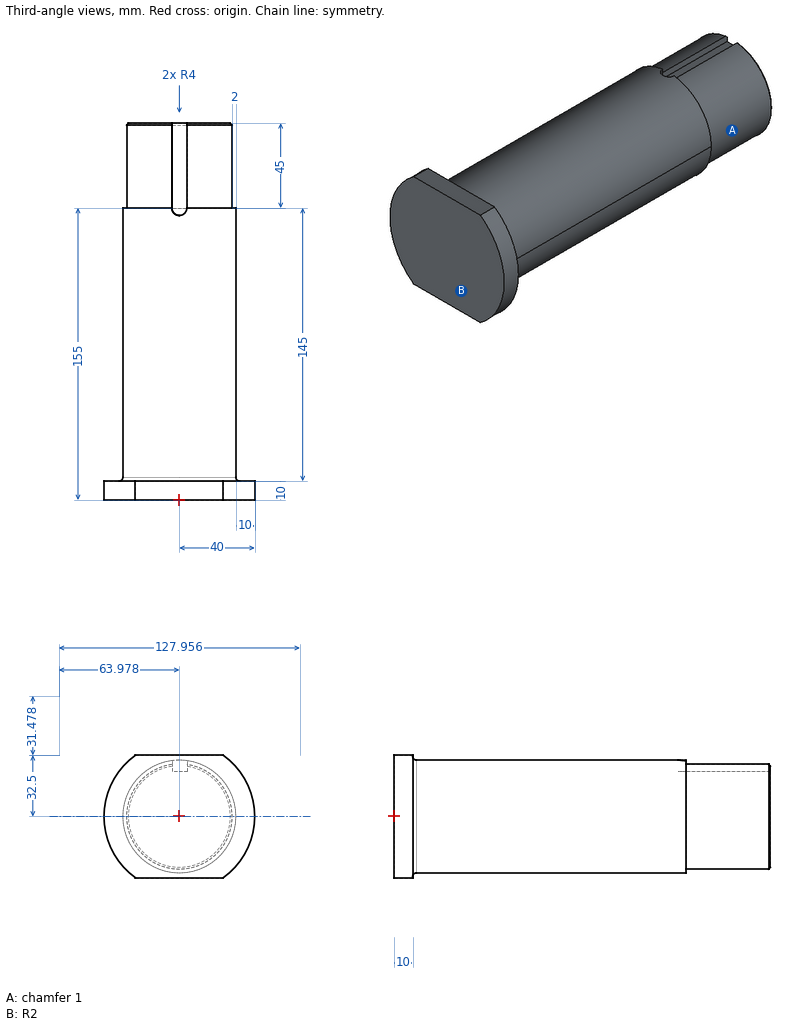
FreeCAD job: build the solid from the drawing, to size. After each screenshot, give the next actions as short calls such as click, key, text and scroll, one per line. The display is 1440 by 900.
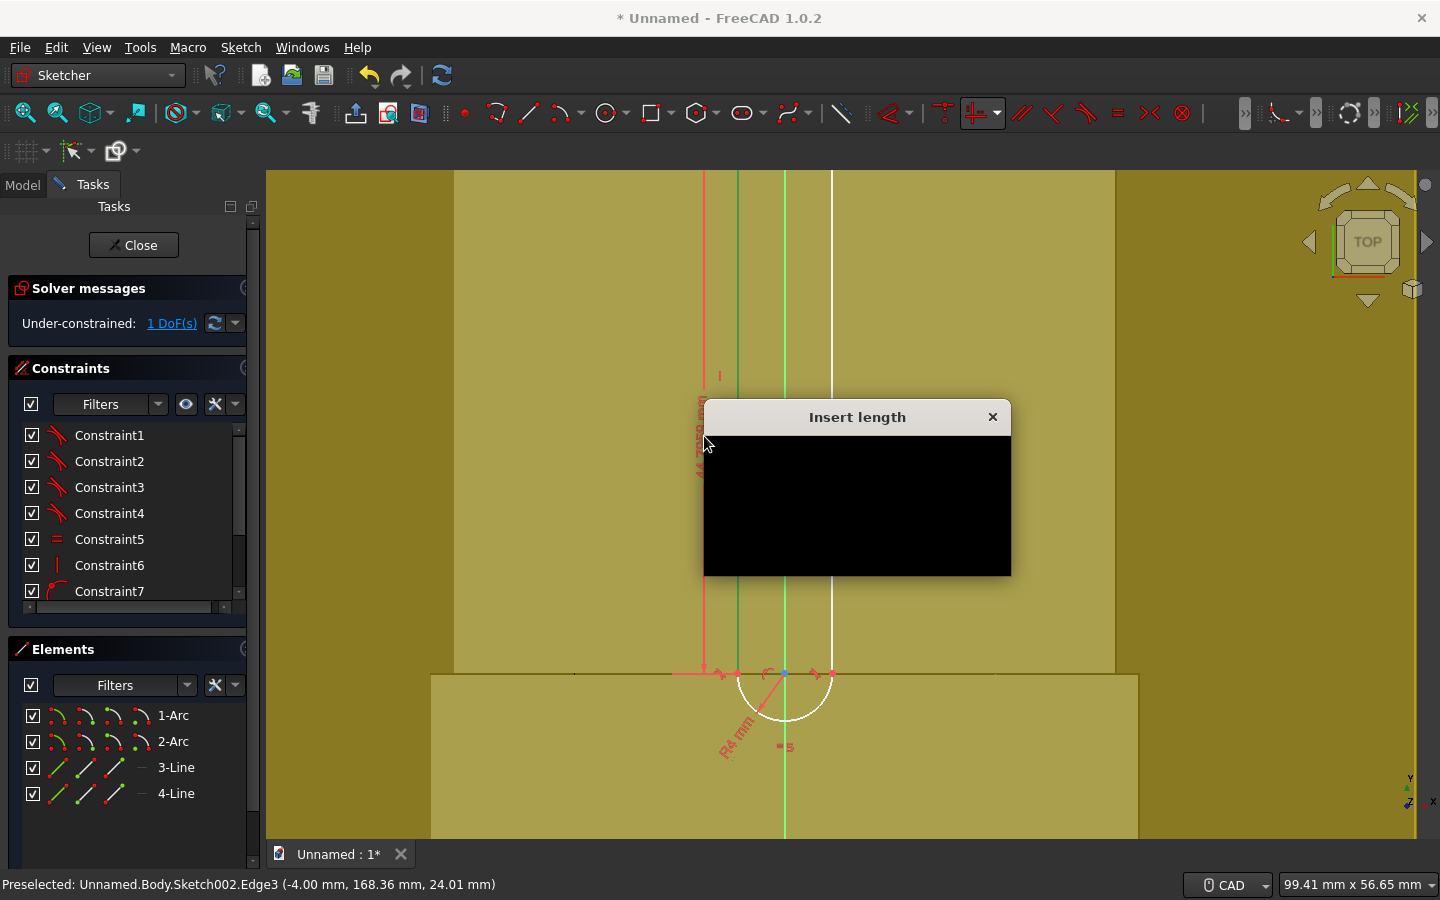
text(45)
key(Return)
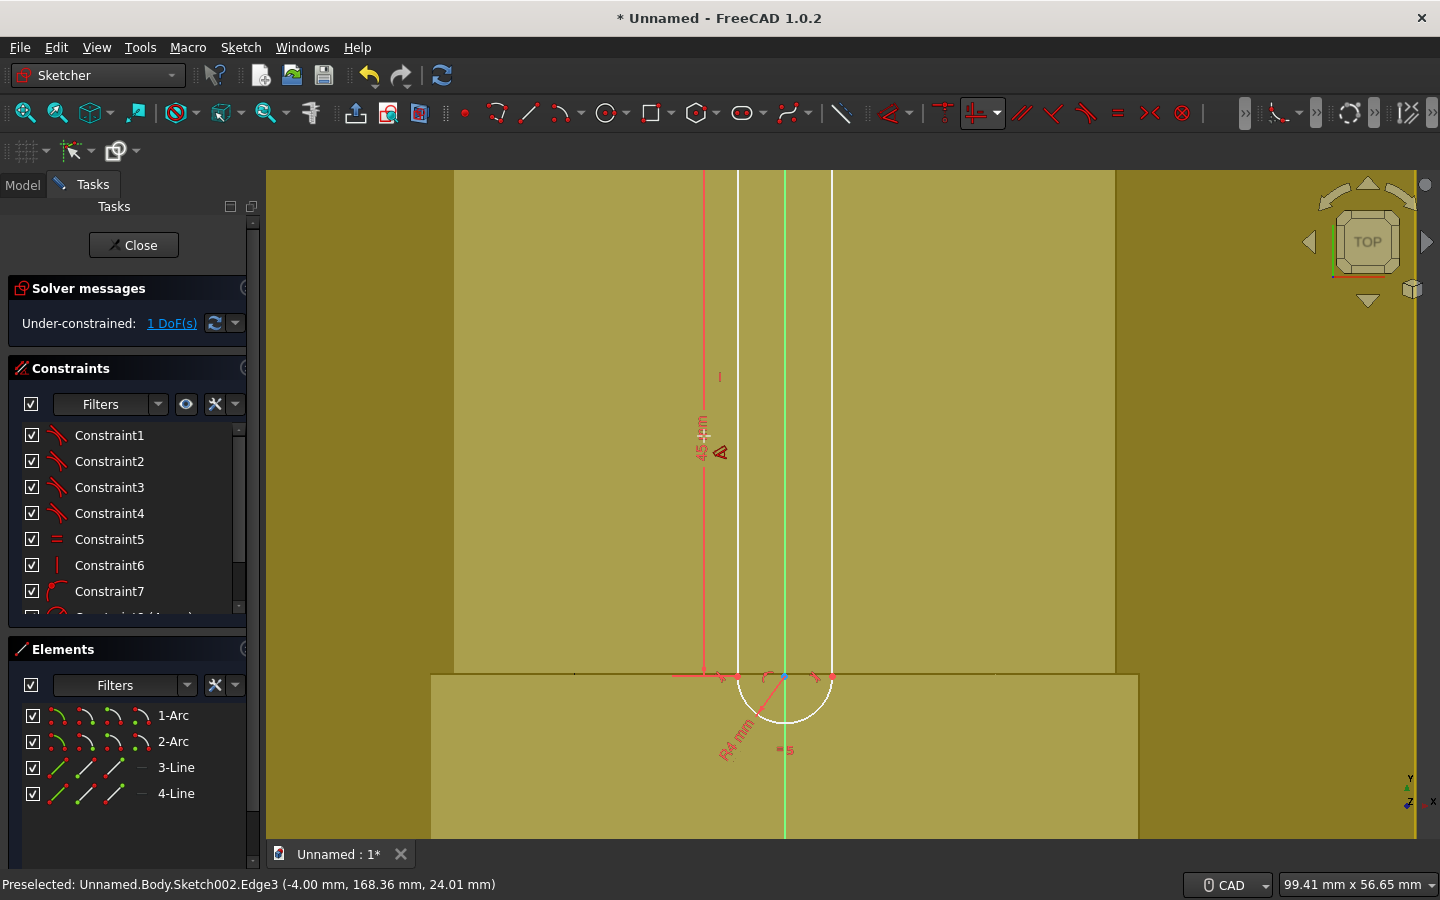
click(738, 676)
click(704, 775)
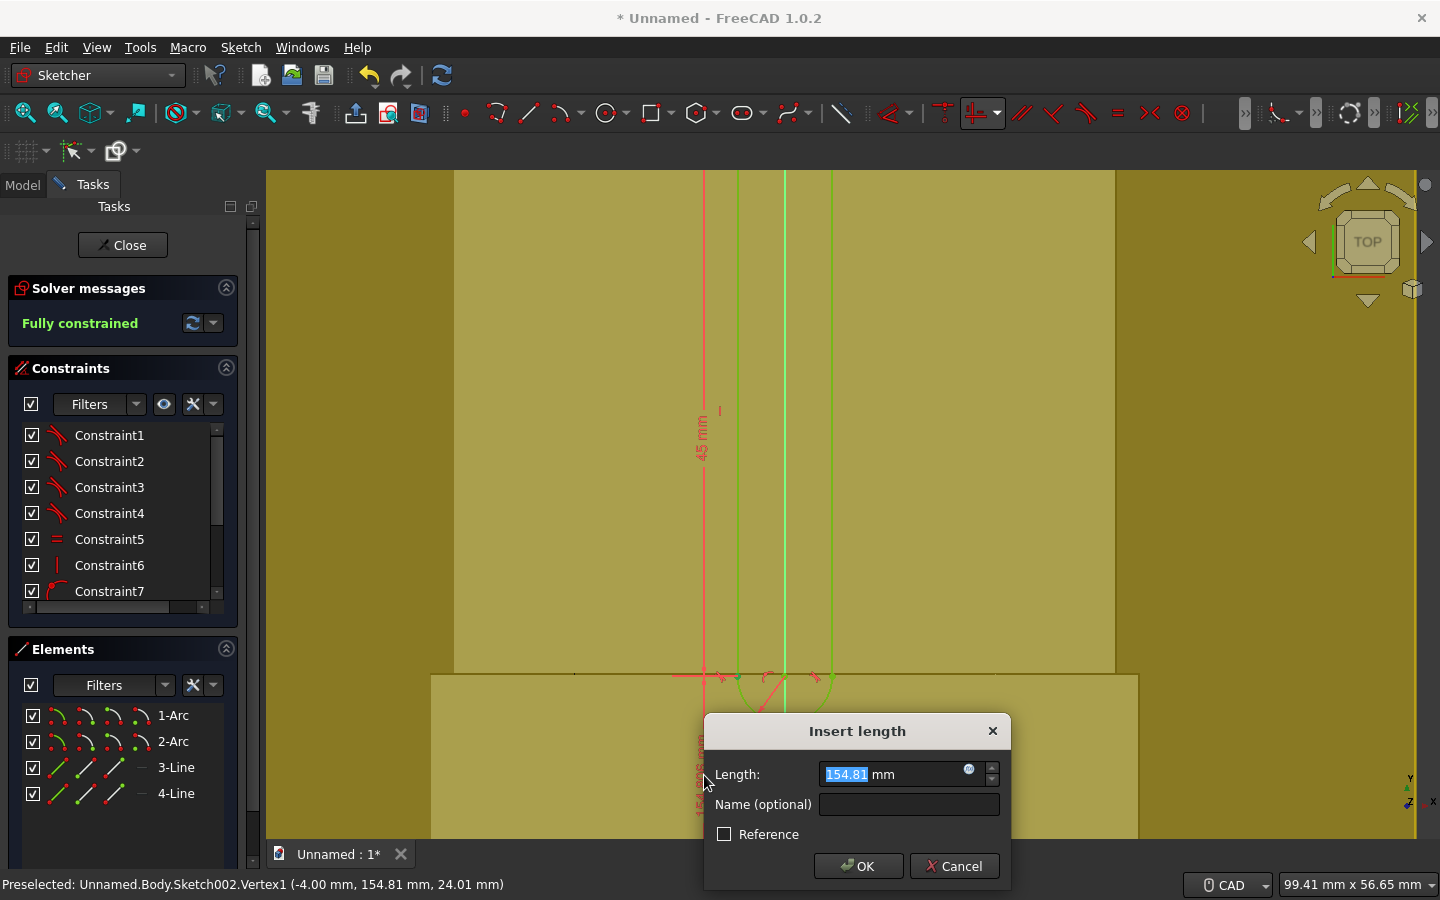
text(155)
key(Return)
key(Escape)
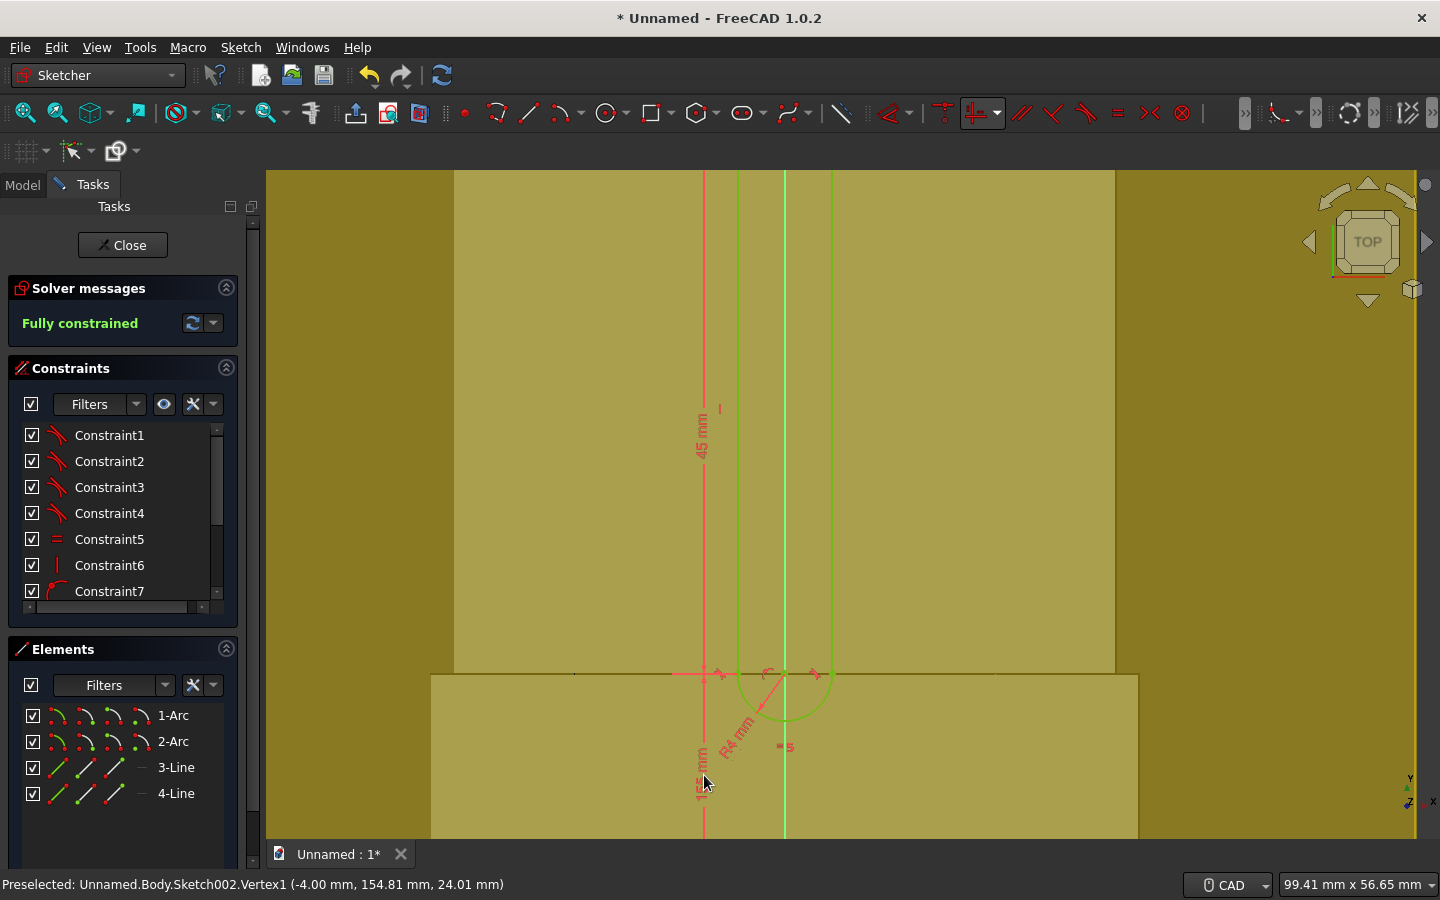
click(123, 245)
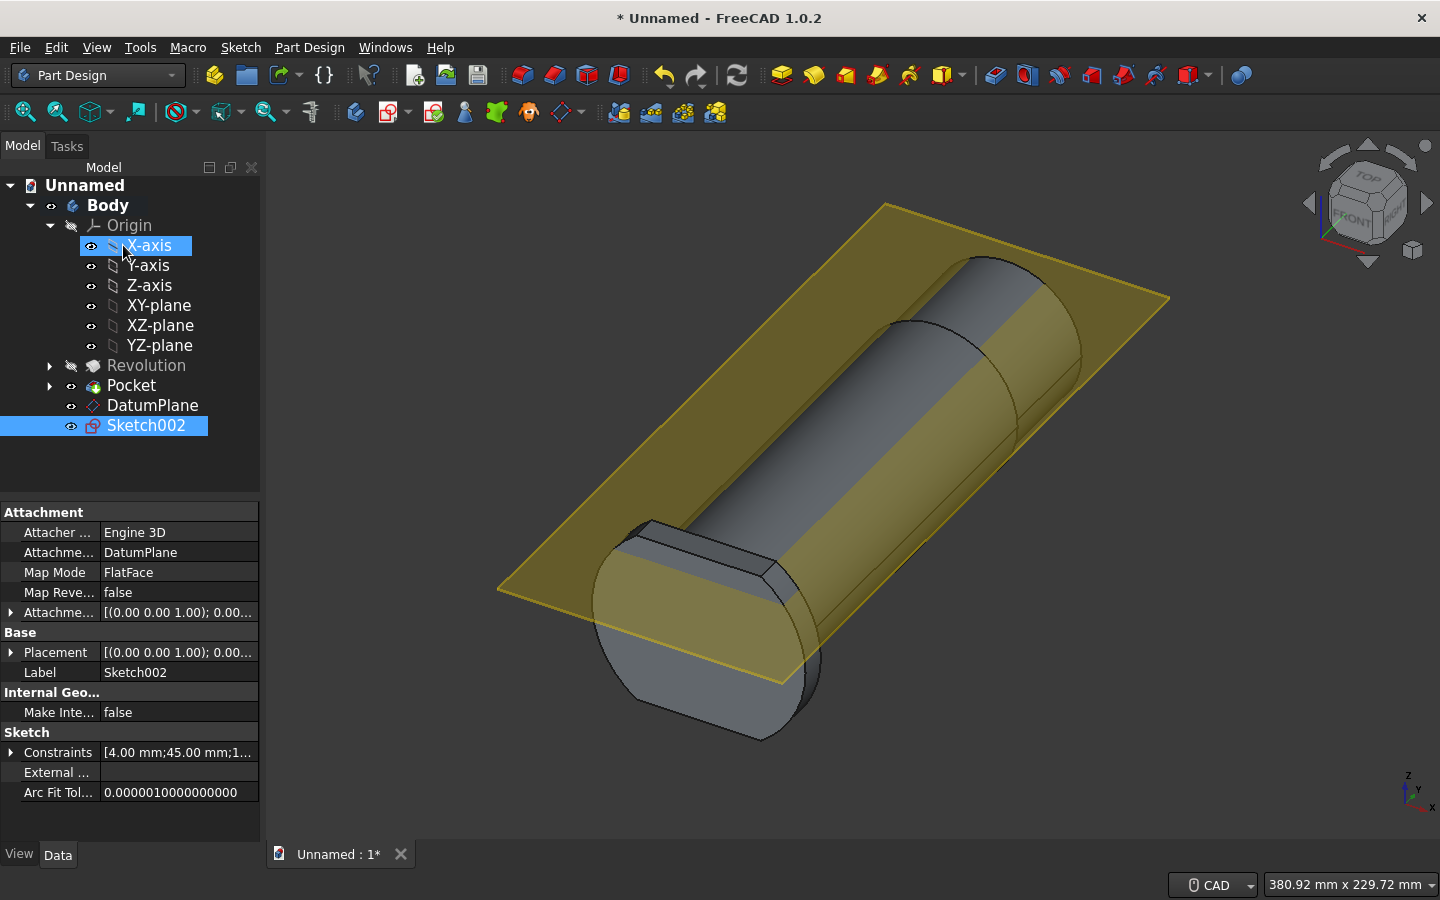
click(996, 76)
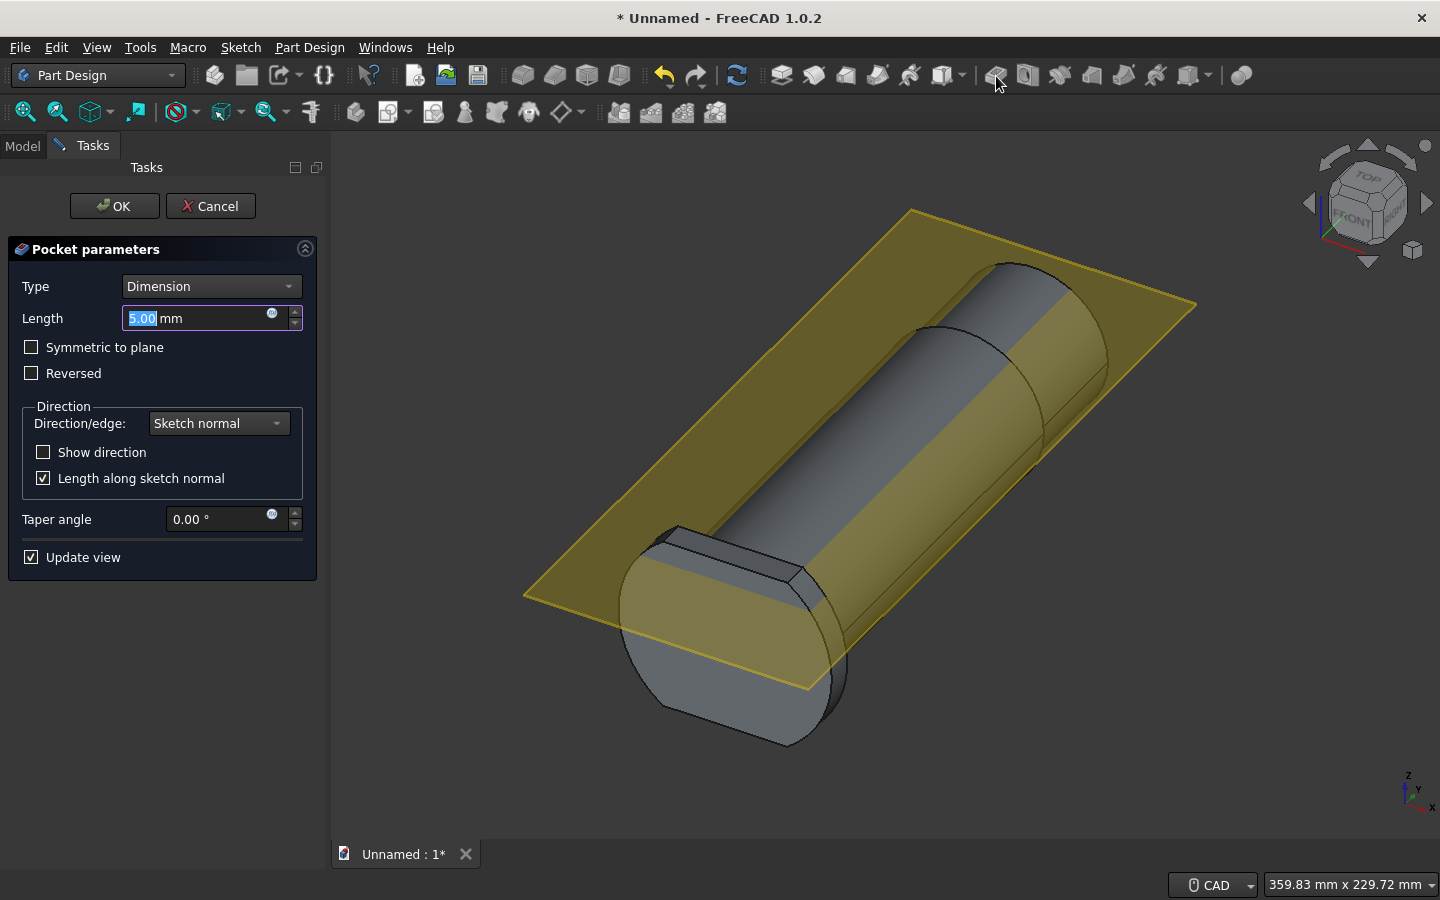
click(212, 286)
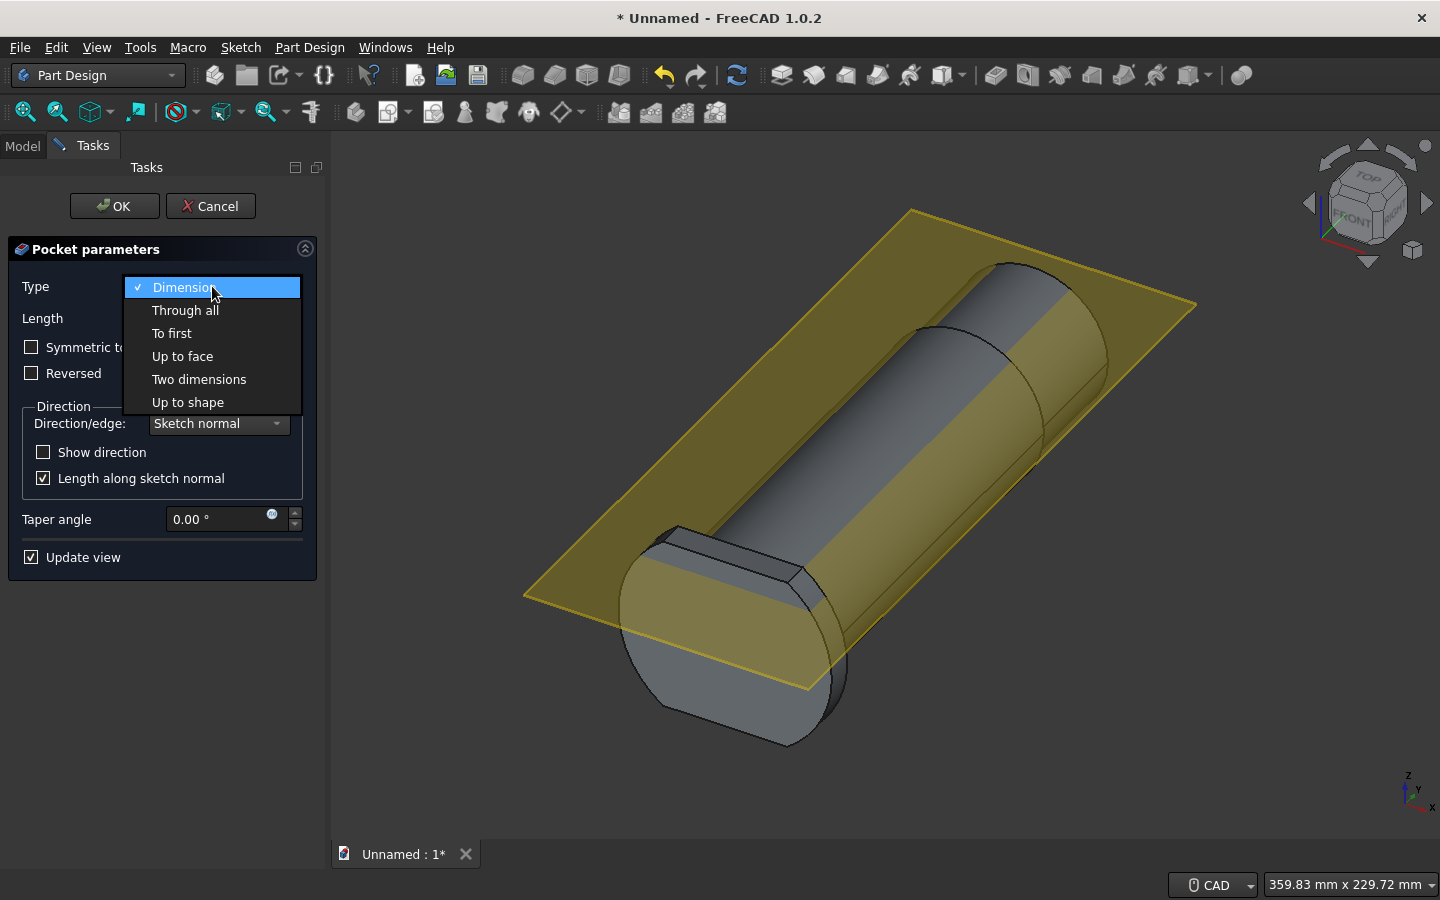
click(212, 334)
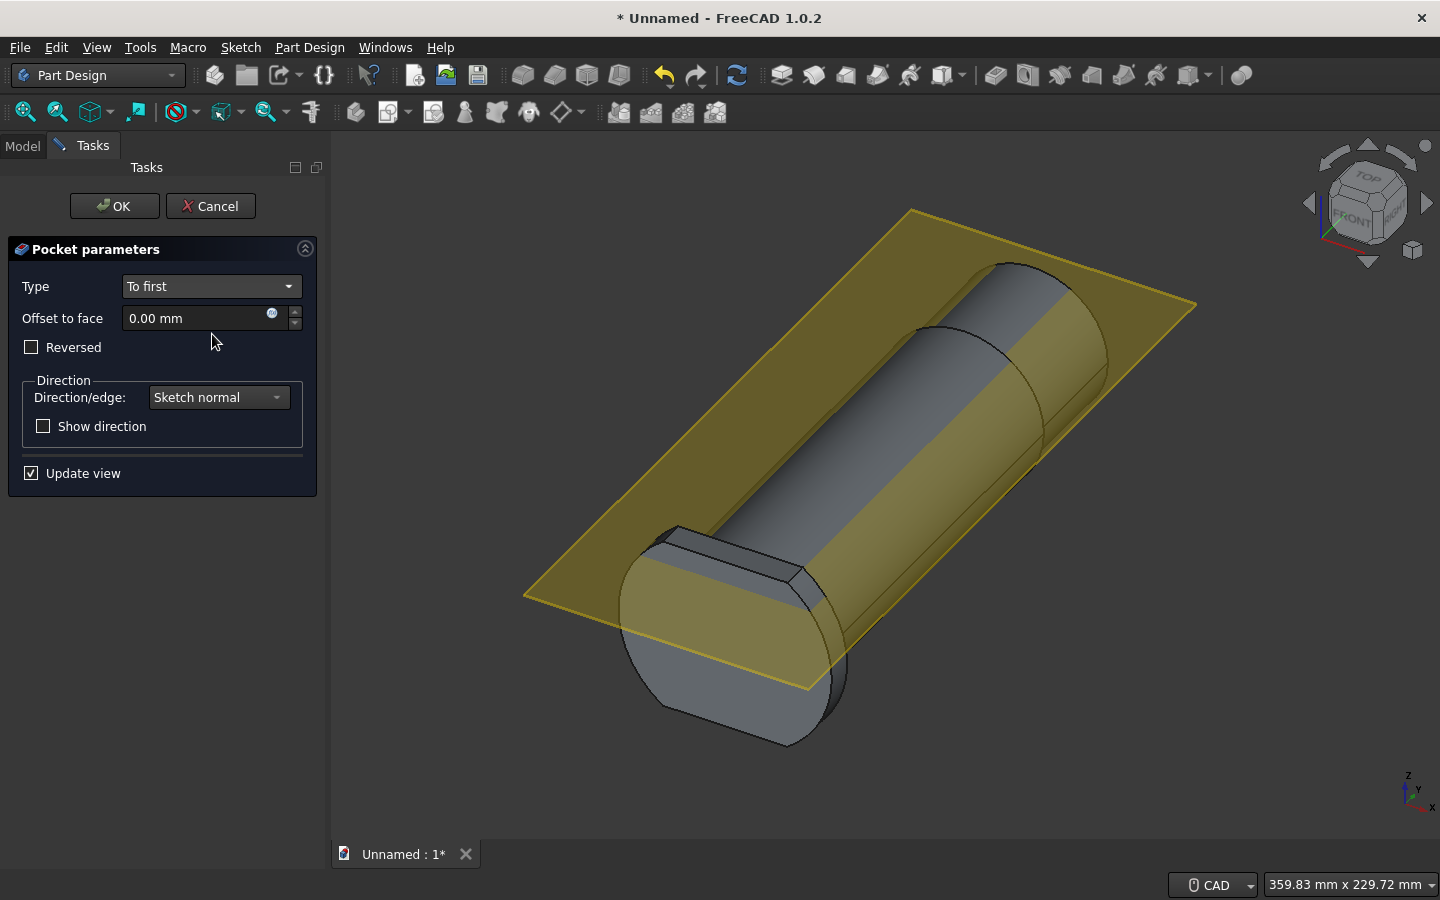
click(30, 347)